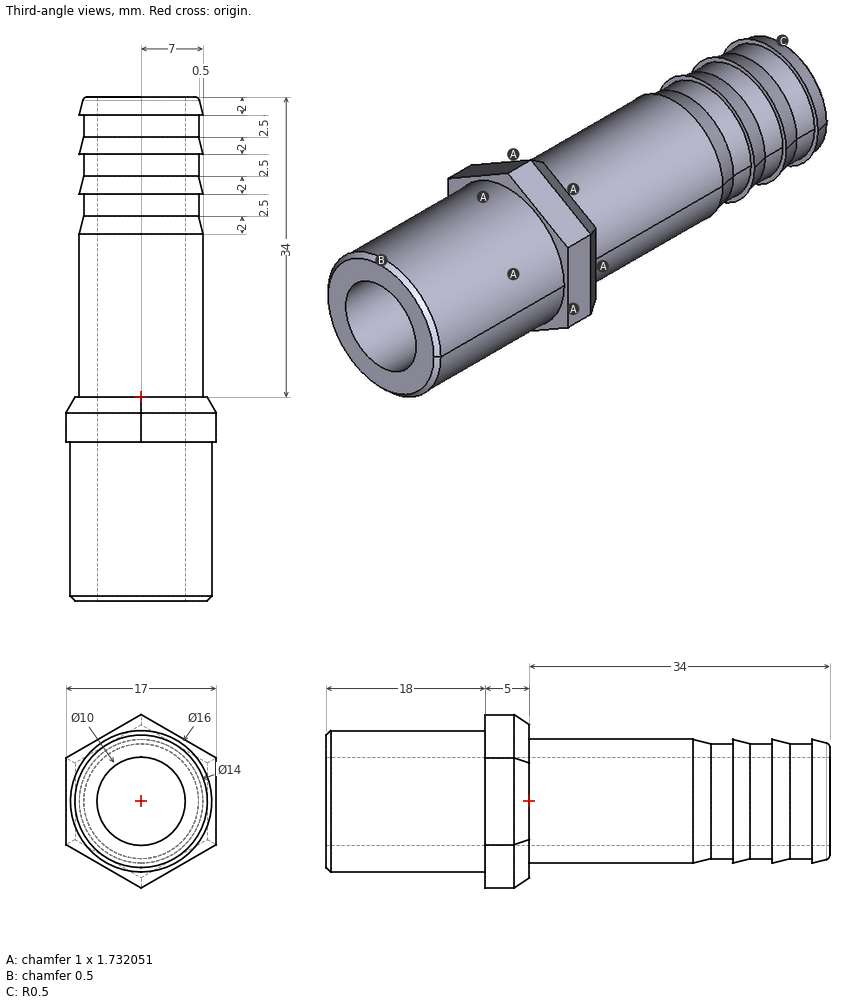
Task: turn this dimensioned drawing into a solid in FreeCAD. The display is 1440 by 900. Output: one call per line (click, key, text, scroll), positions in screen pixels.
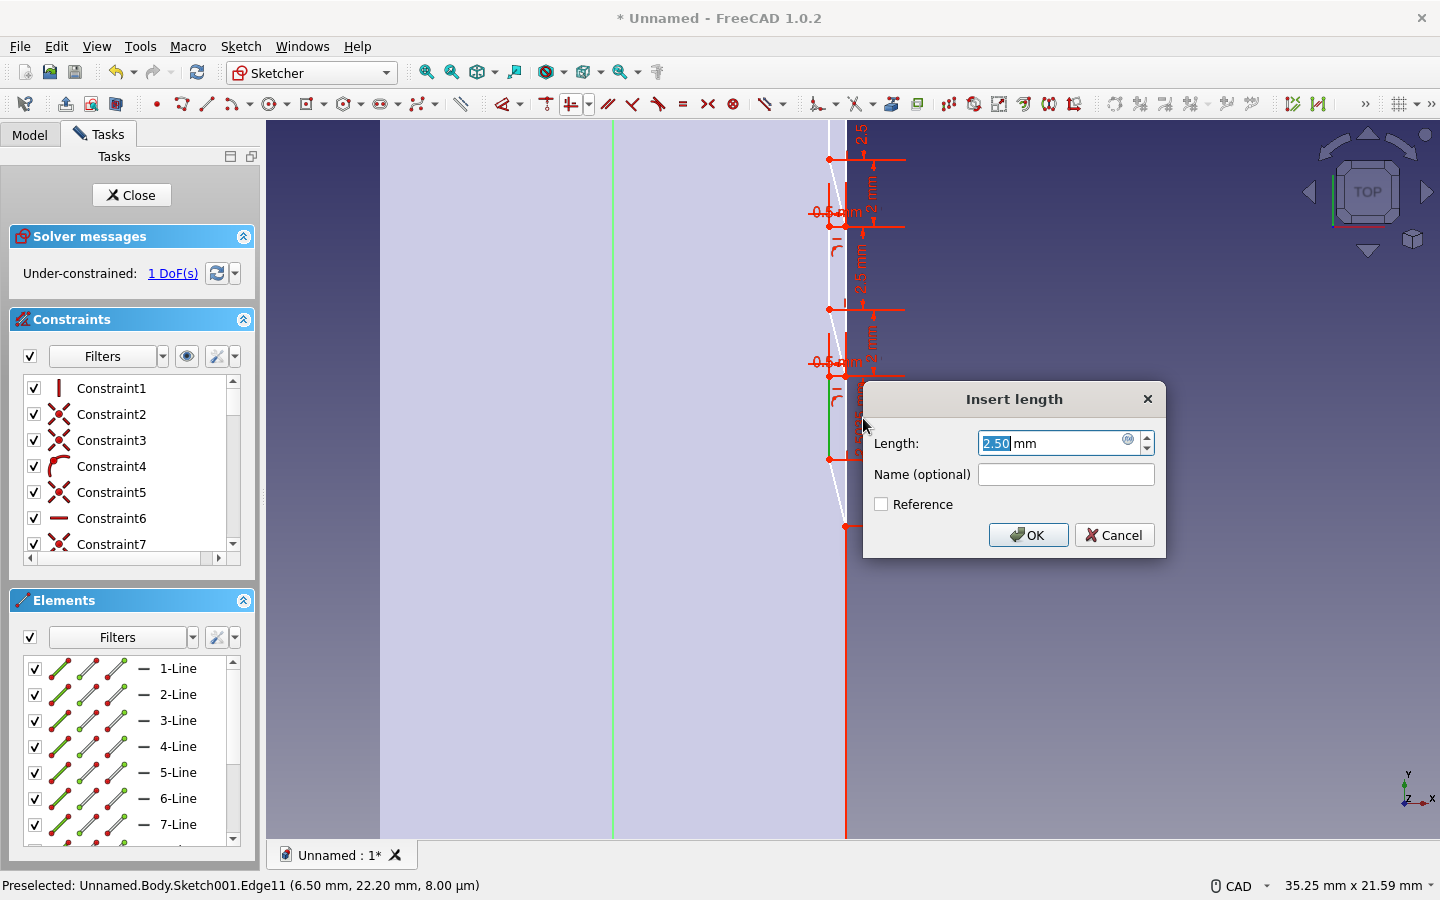
text(2.5)
key(Return)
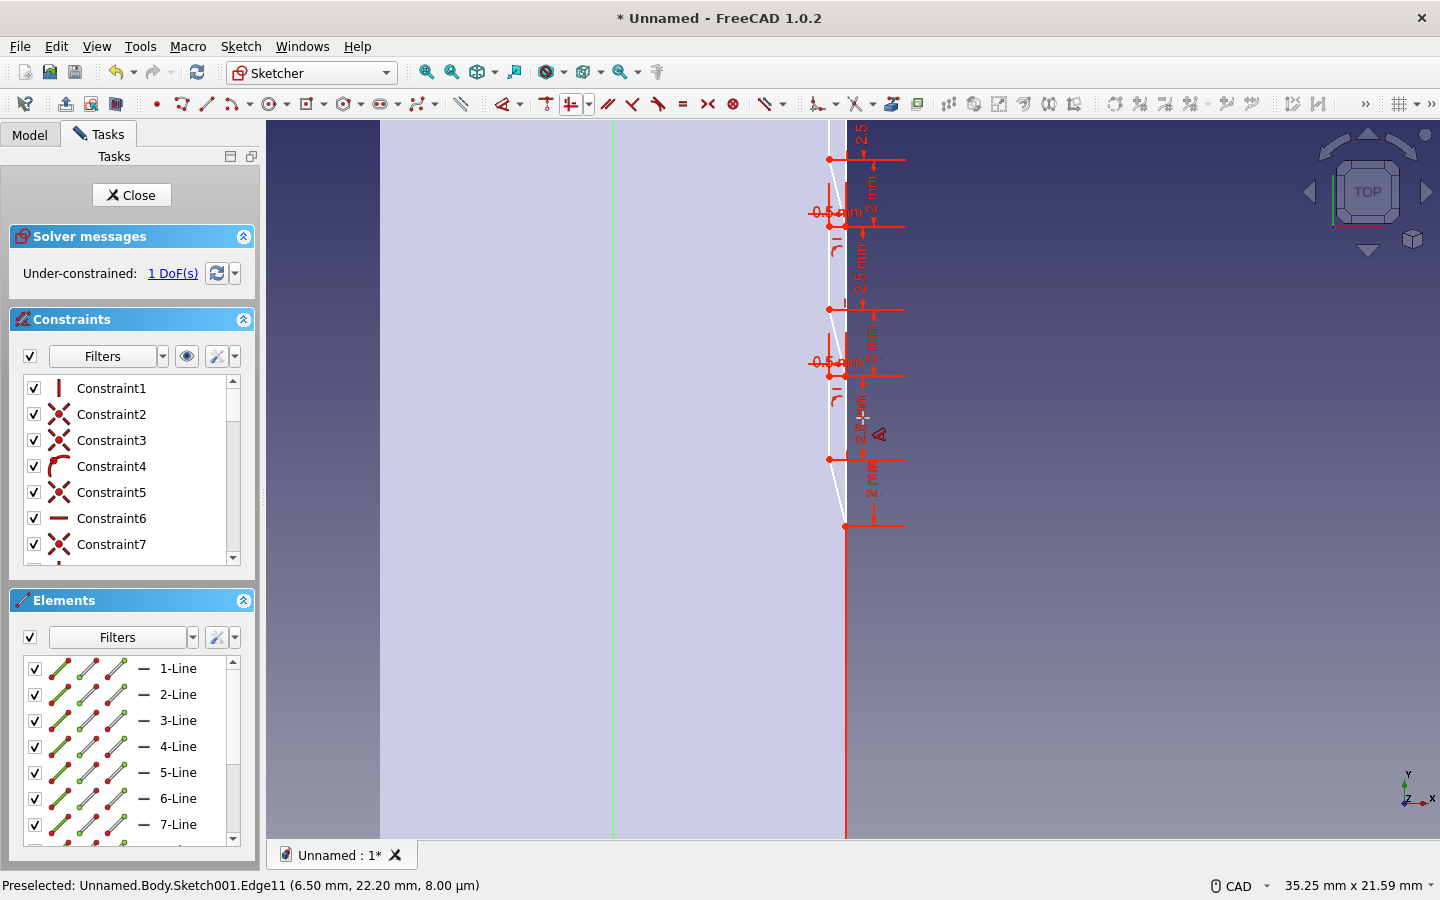
scroll(829, 402, down, 4)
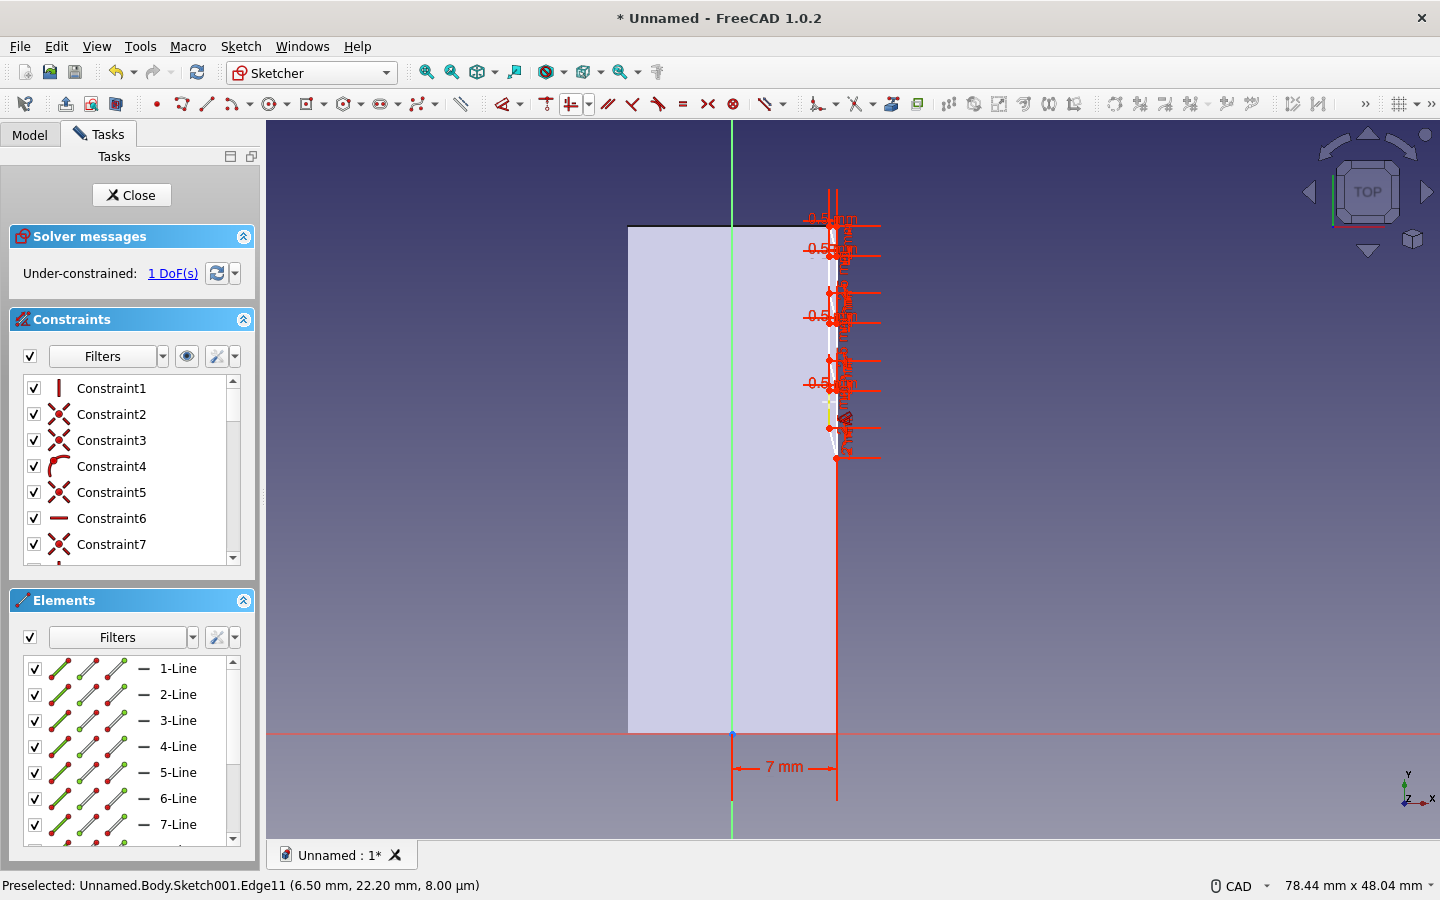
scroll(837, 226, up, 3)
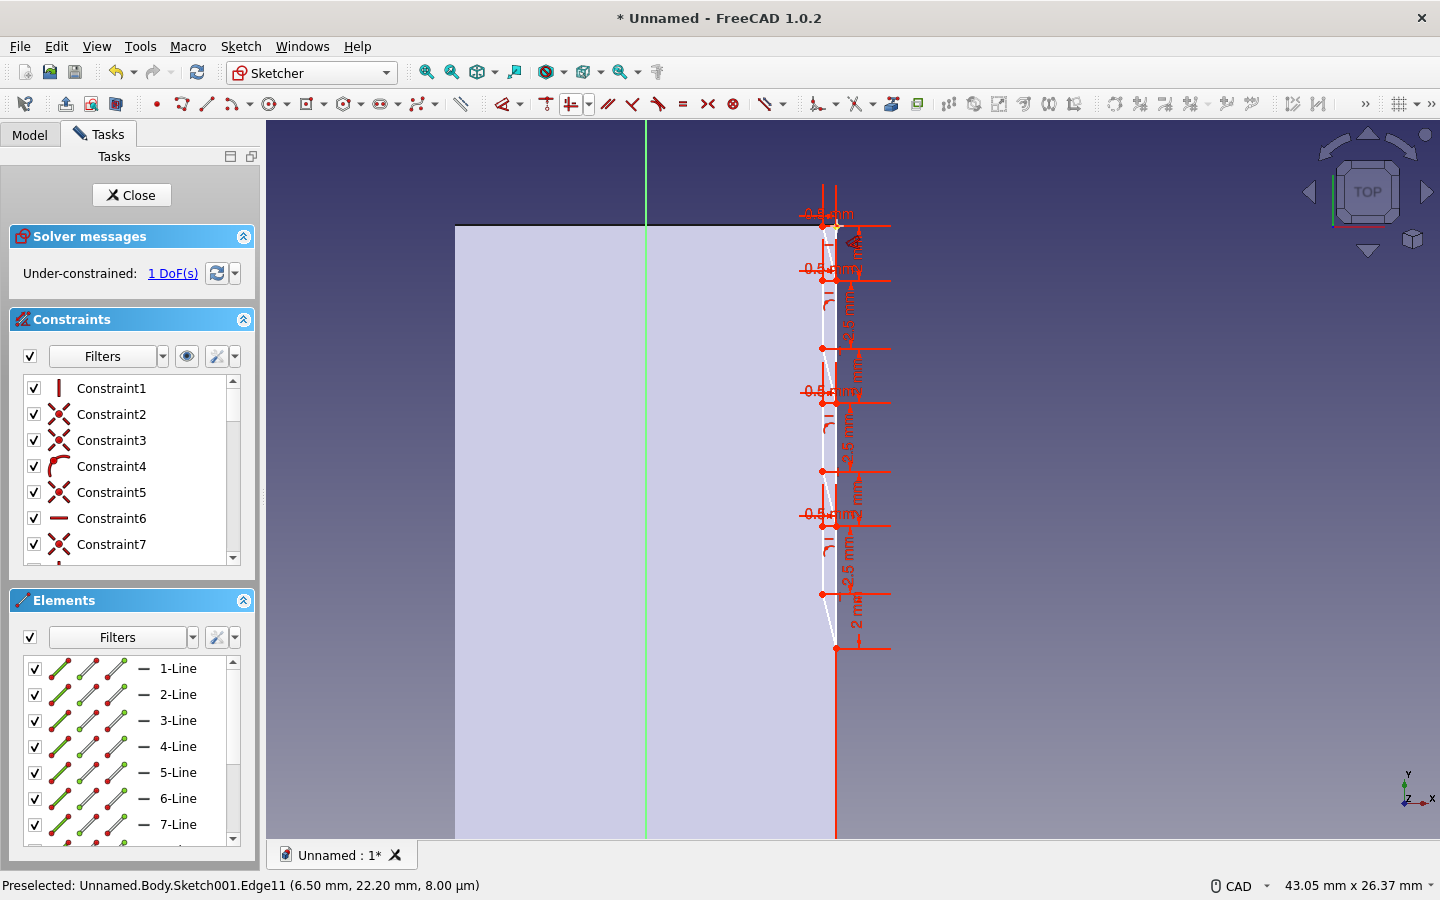
click(836, 226)
click(870, 653)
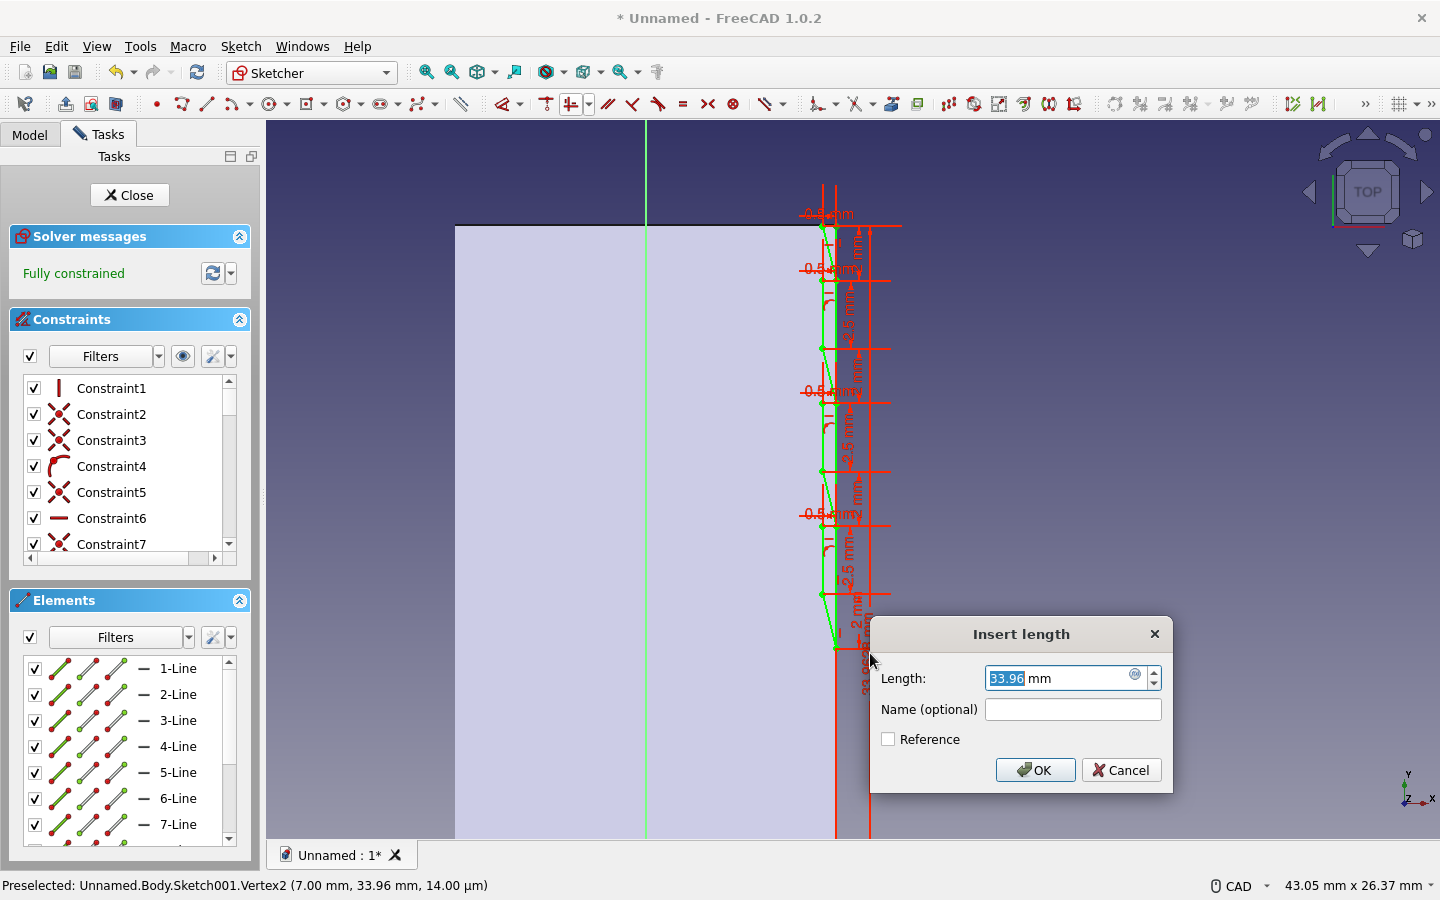
text(34)
key(Return)
key(Escape)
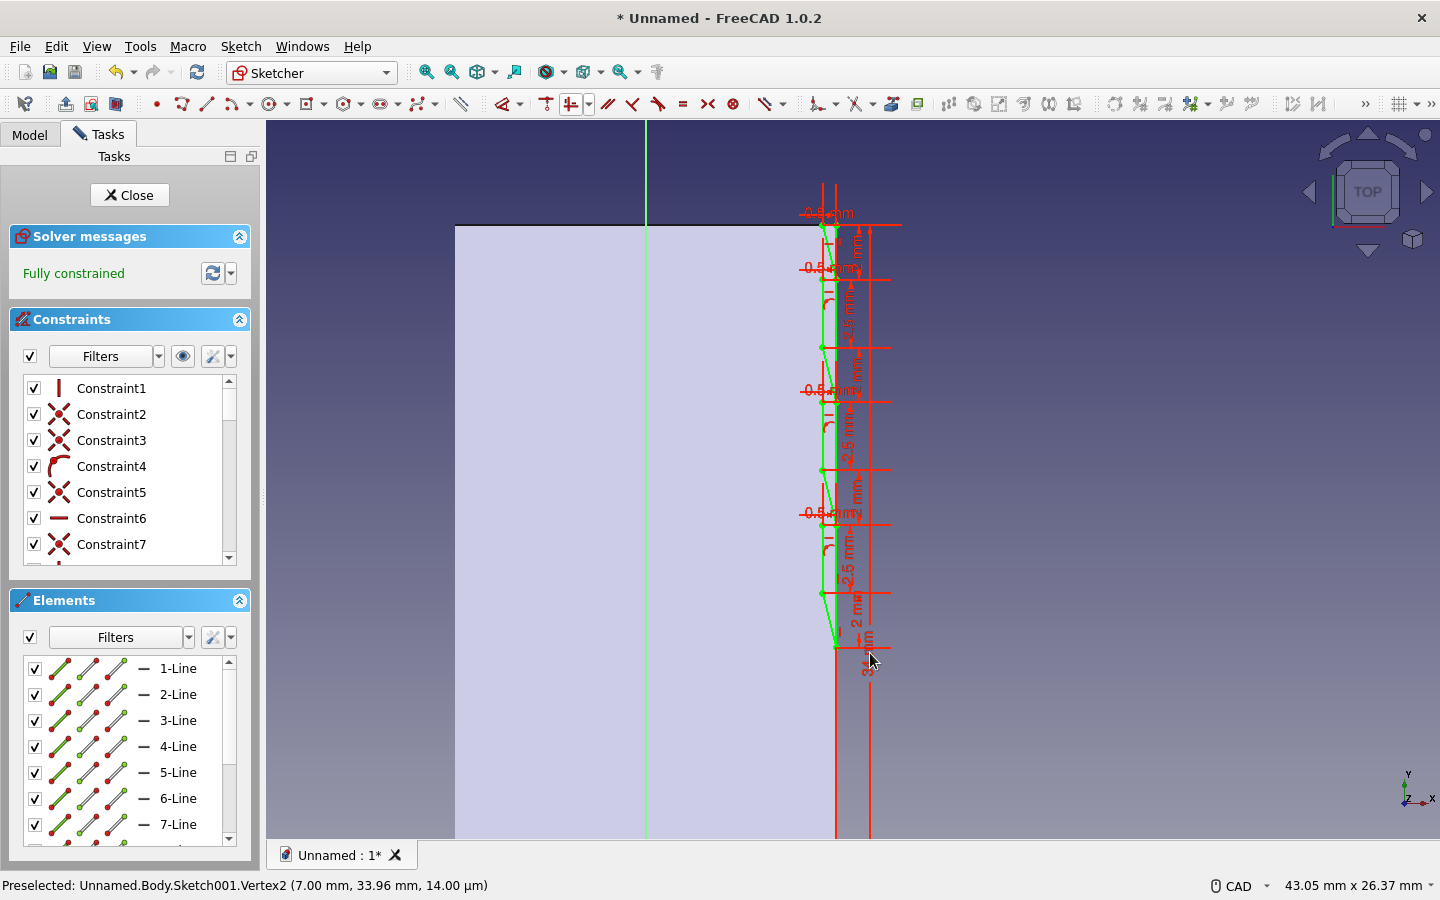
click(130, 195)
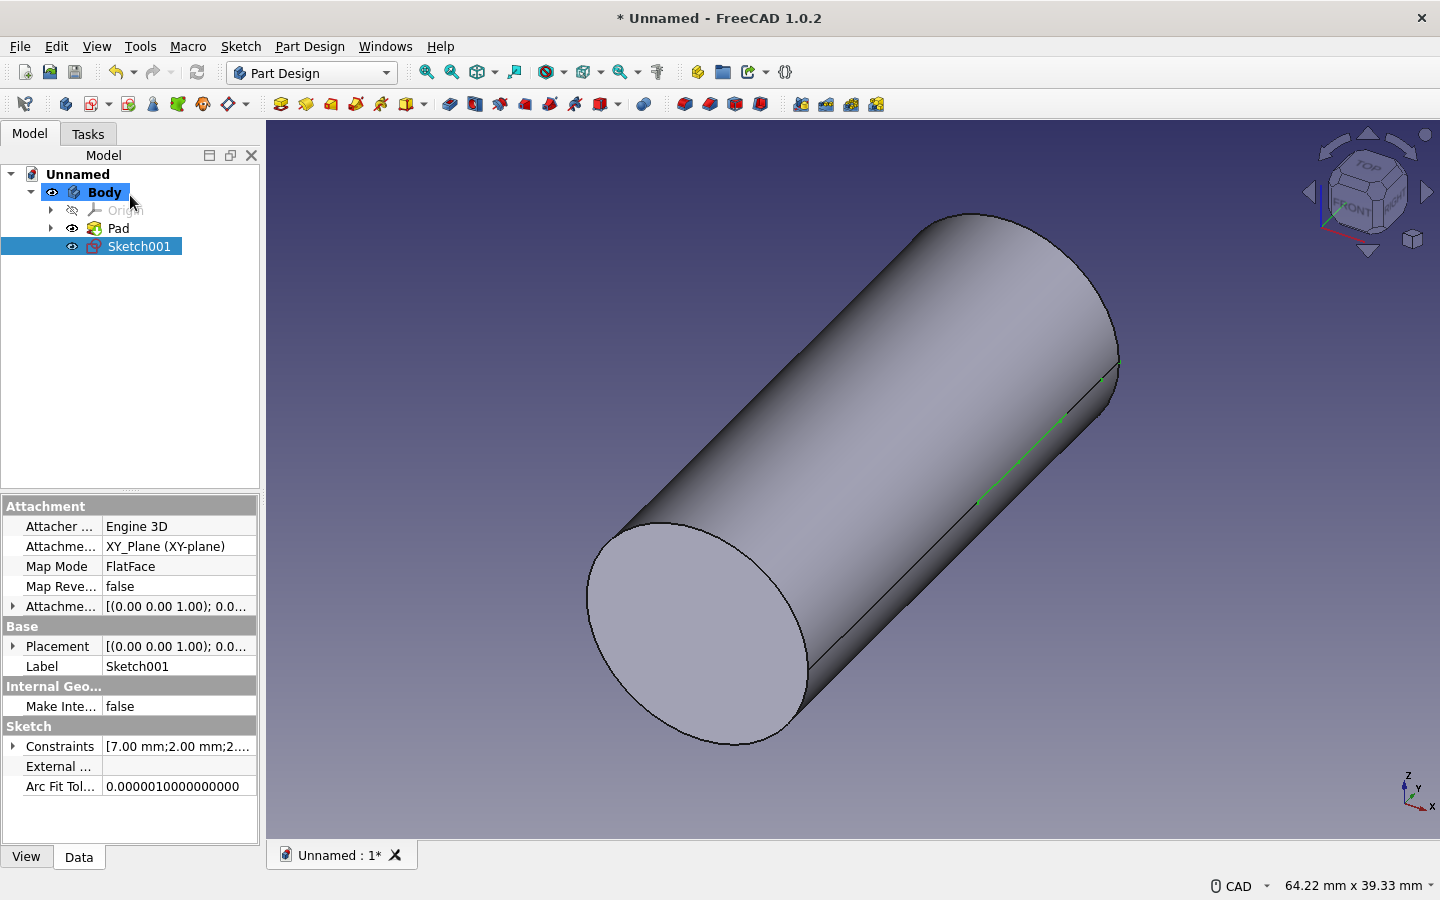
click(500, 104)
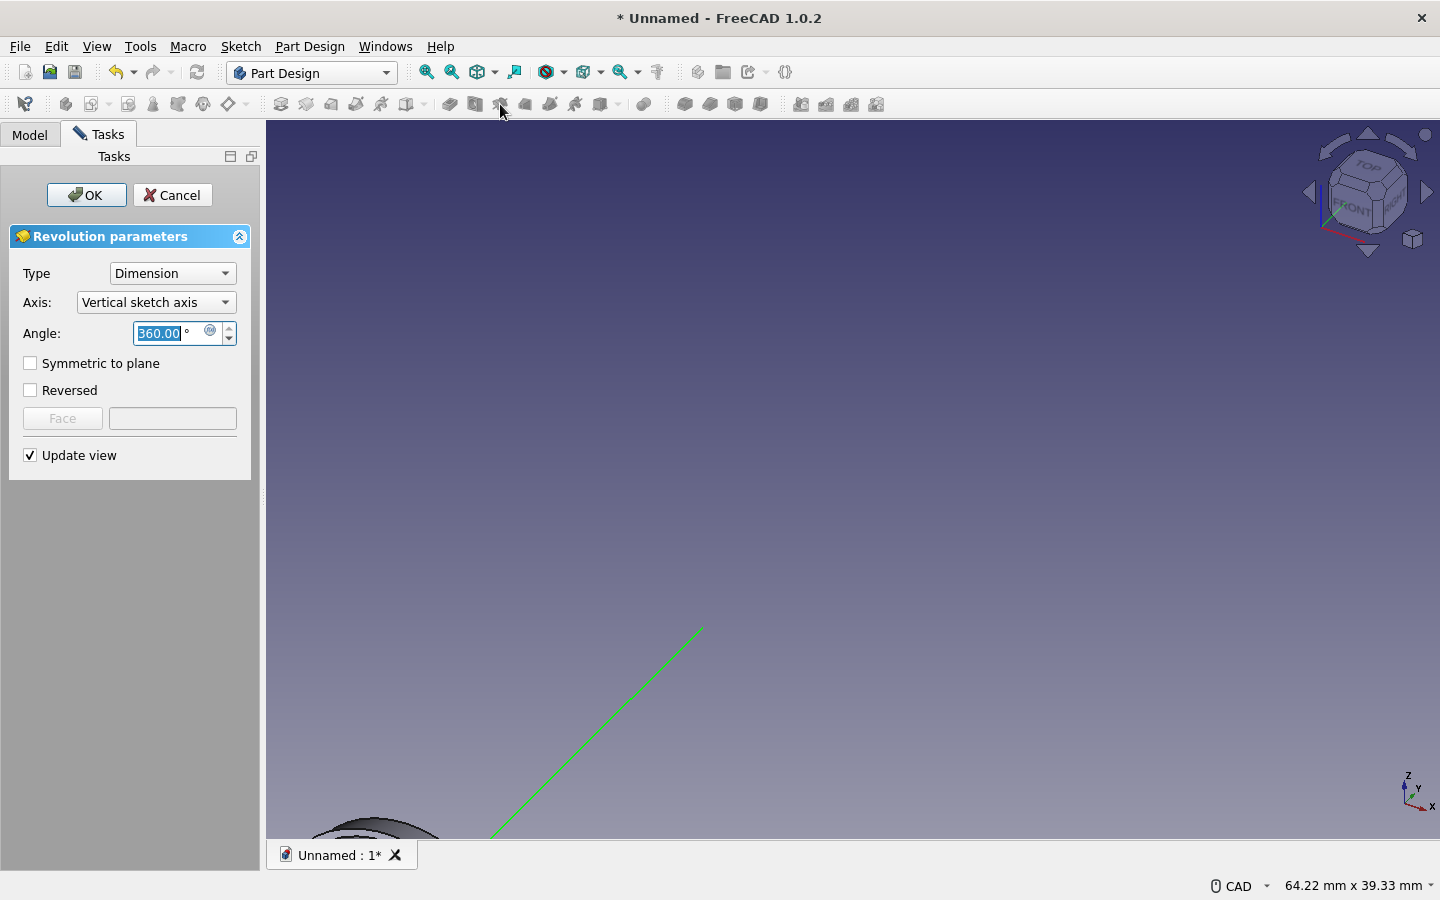
click(87, 195)